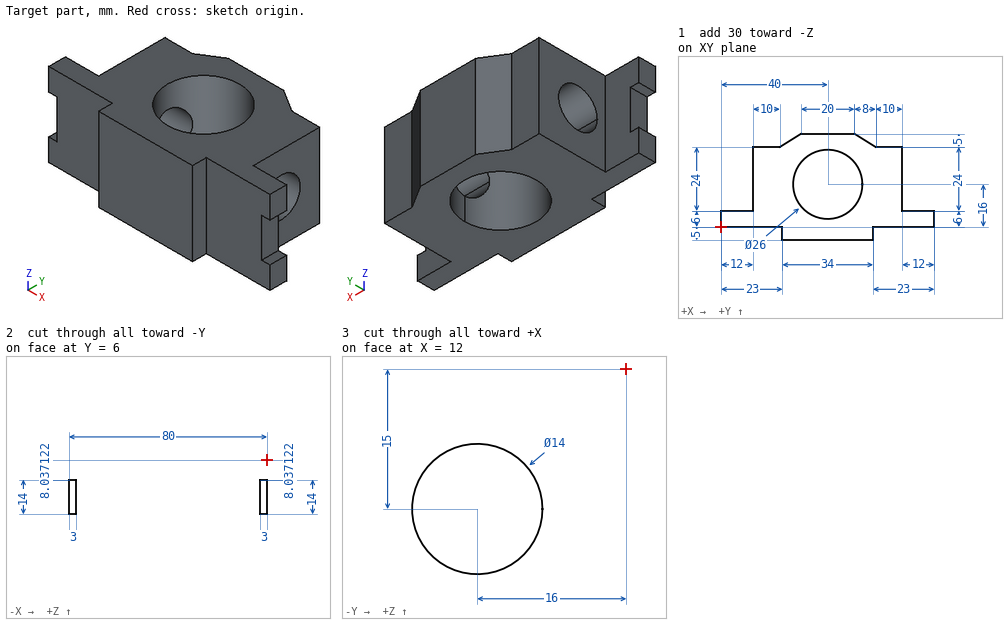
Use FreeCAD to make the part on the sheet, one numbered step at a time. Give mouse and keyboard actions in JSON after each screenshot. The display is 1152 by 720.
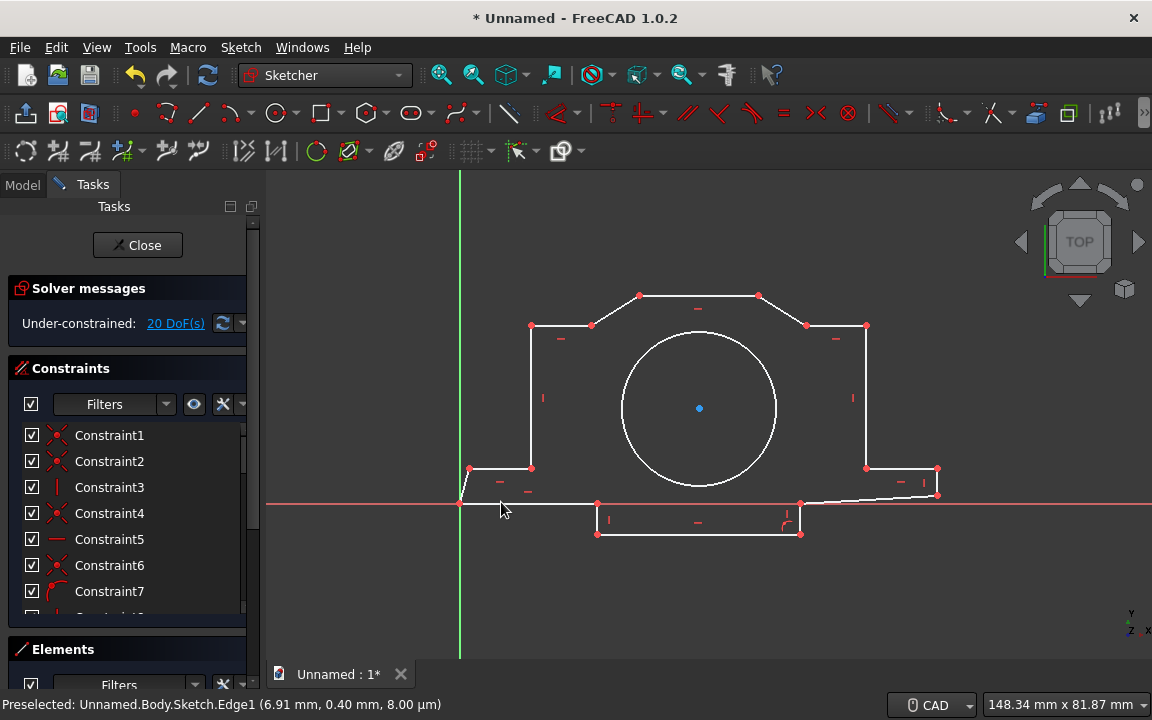
{"action": "left_click", "coordinate": [841, 502]}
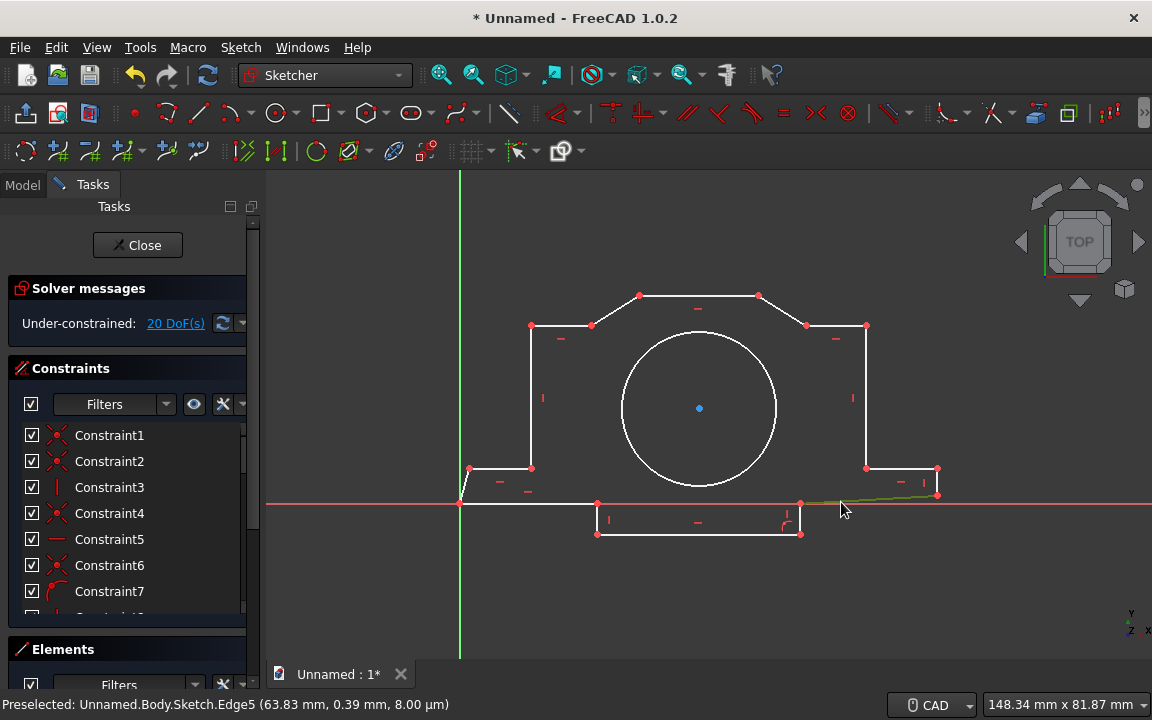
{"action": "key", "text": "h"}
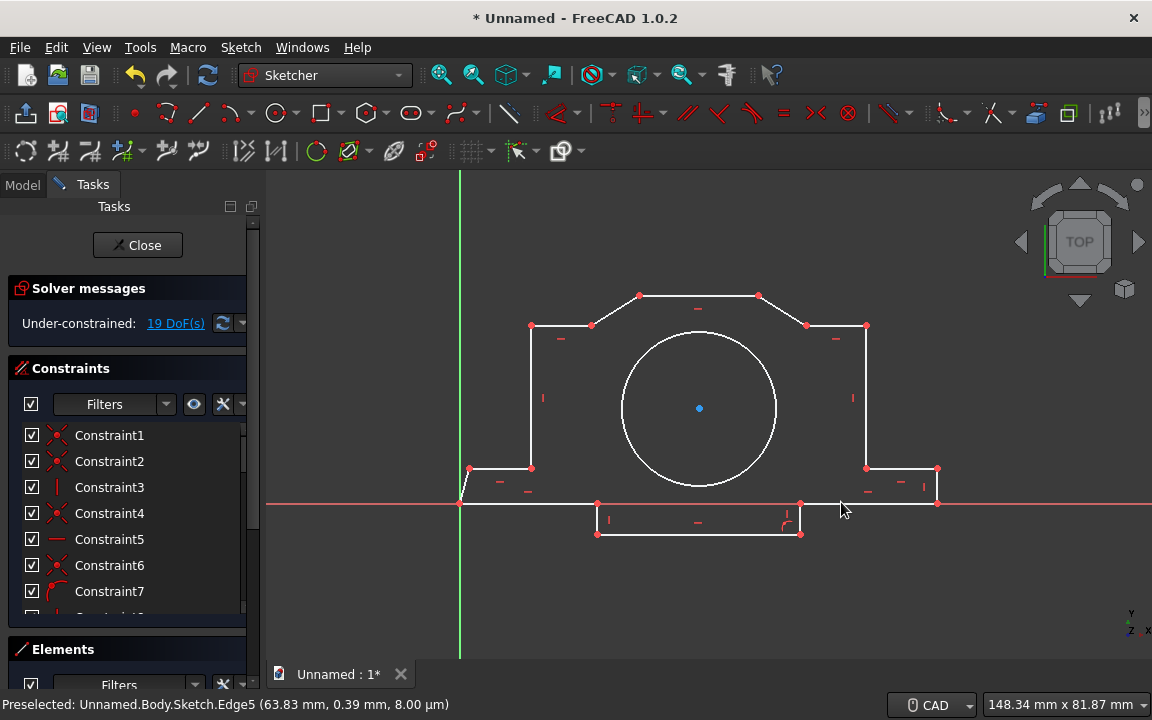
{"action": "scroll", "coordinate": [462, 493], "scroll_direction": "up", "scroll_amount": 2}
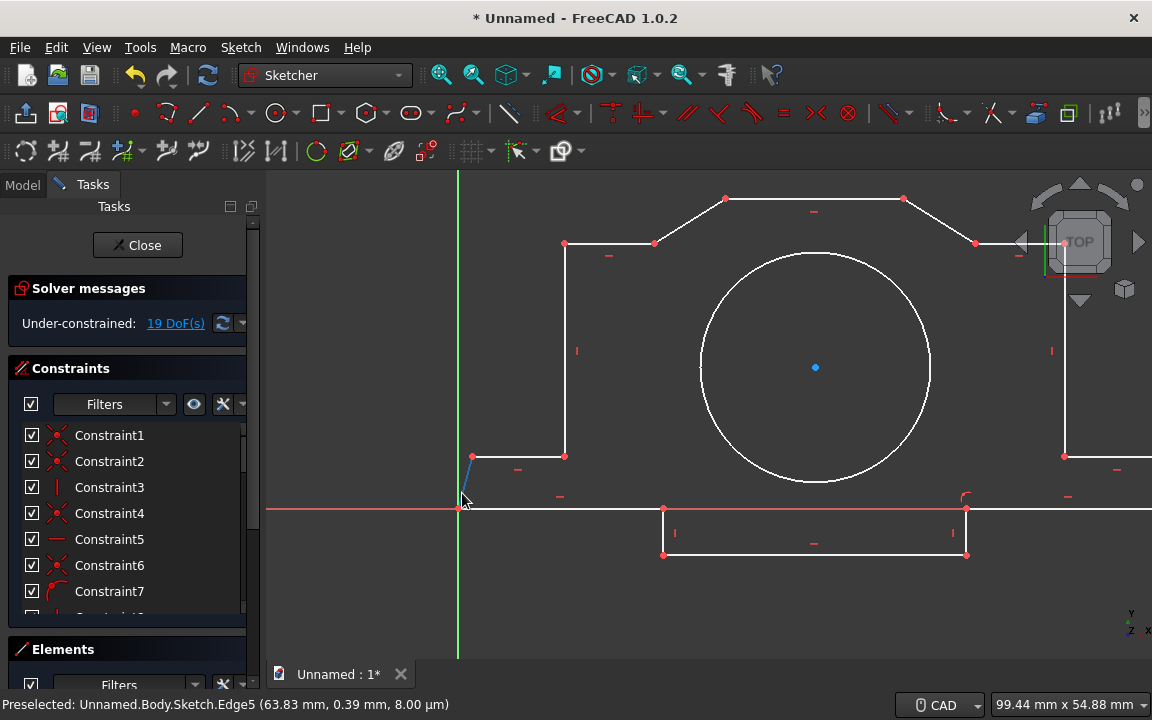
{"action": "left_click", "coordinate": [463, 493]}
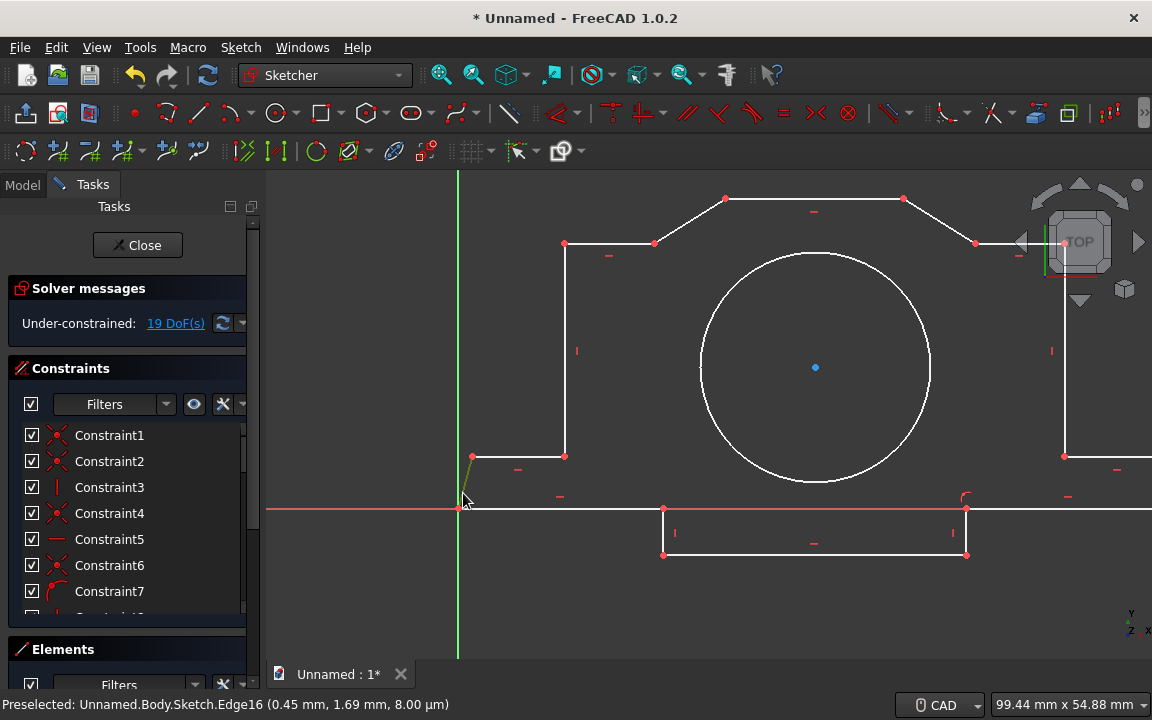
{"action": "key", "text": "v"}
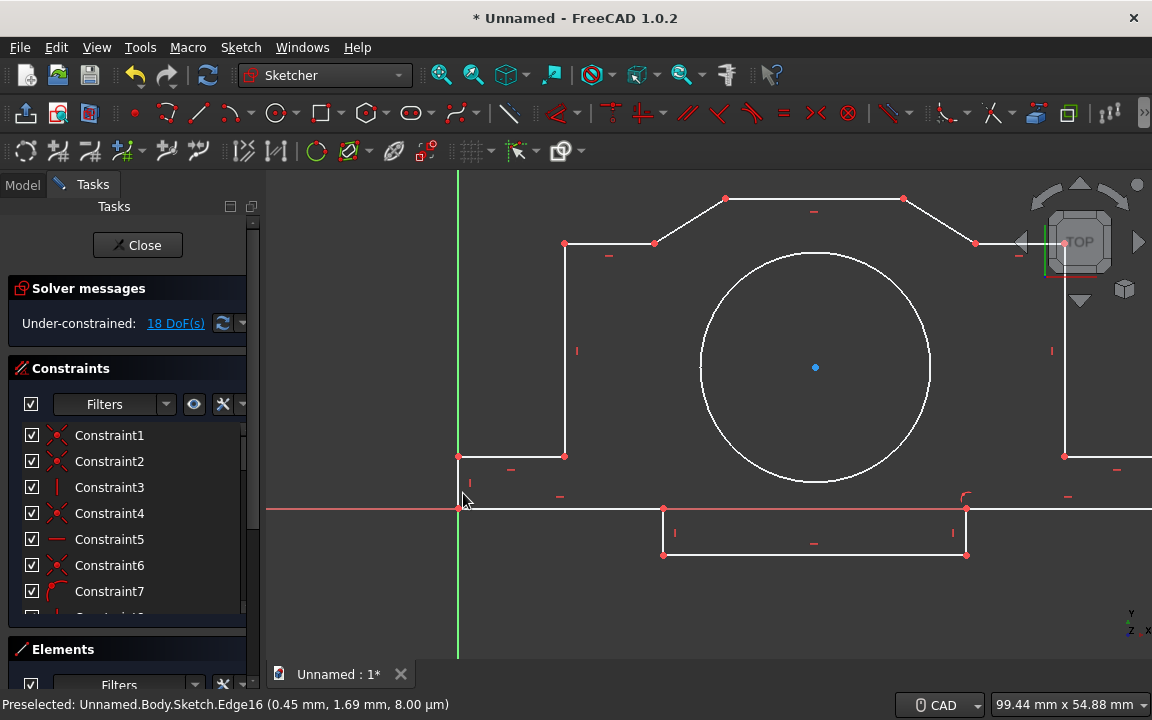
{"action": "left_click", "coordinate": [556, 114]}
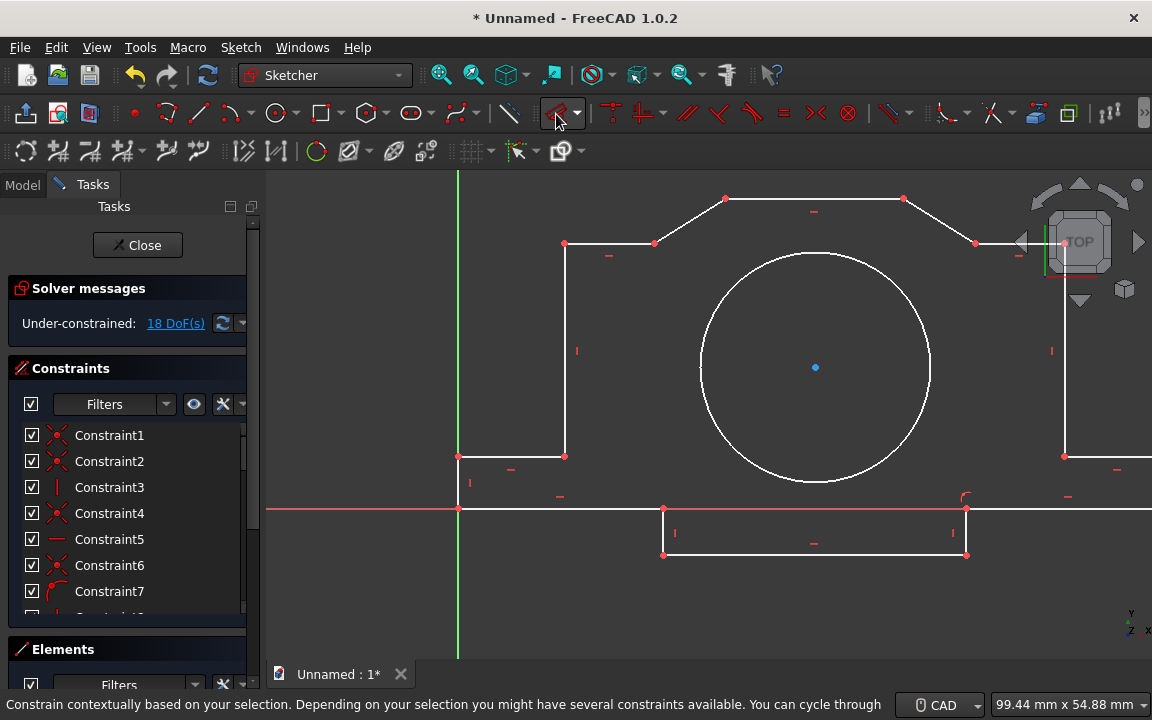
{"action": "left_click", "coordinate": [897, 286]}
{"action": "left_click", "coordinate": [920, 263]}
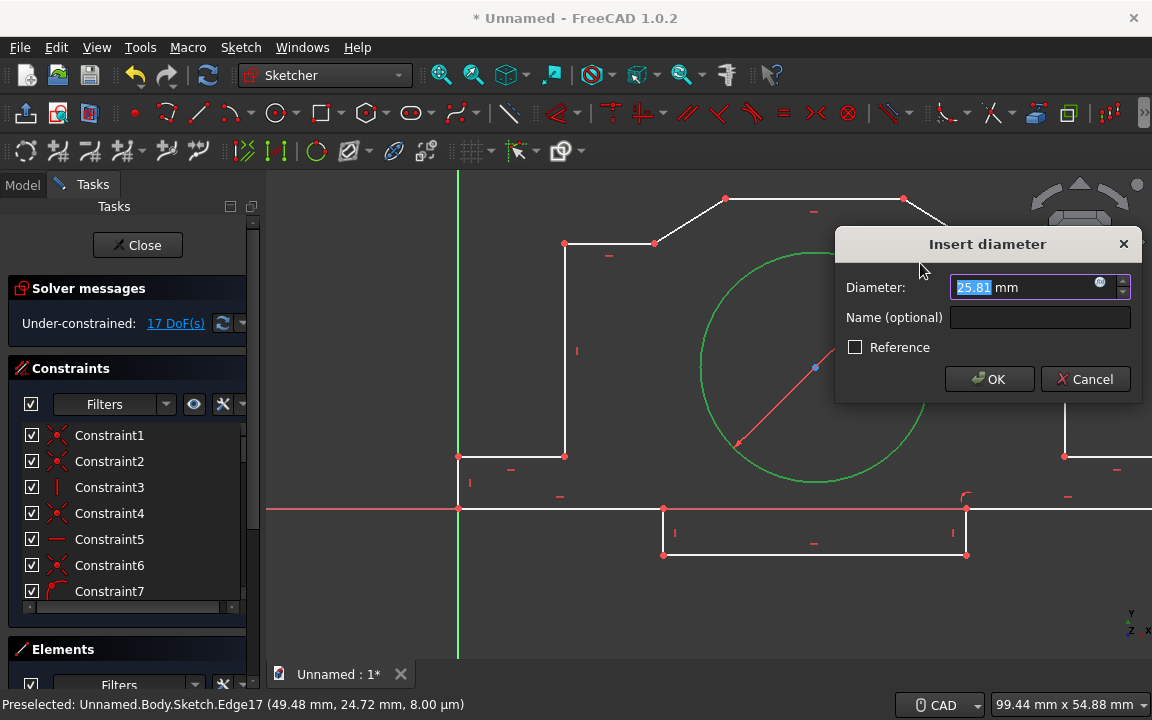
{"action": "type", "text": "26"}
{"action": "key", "text": "Return"}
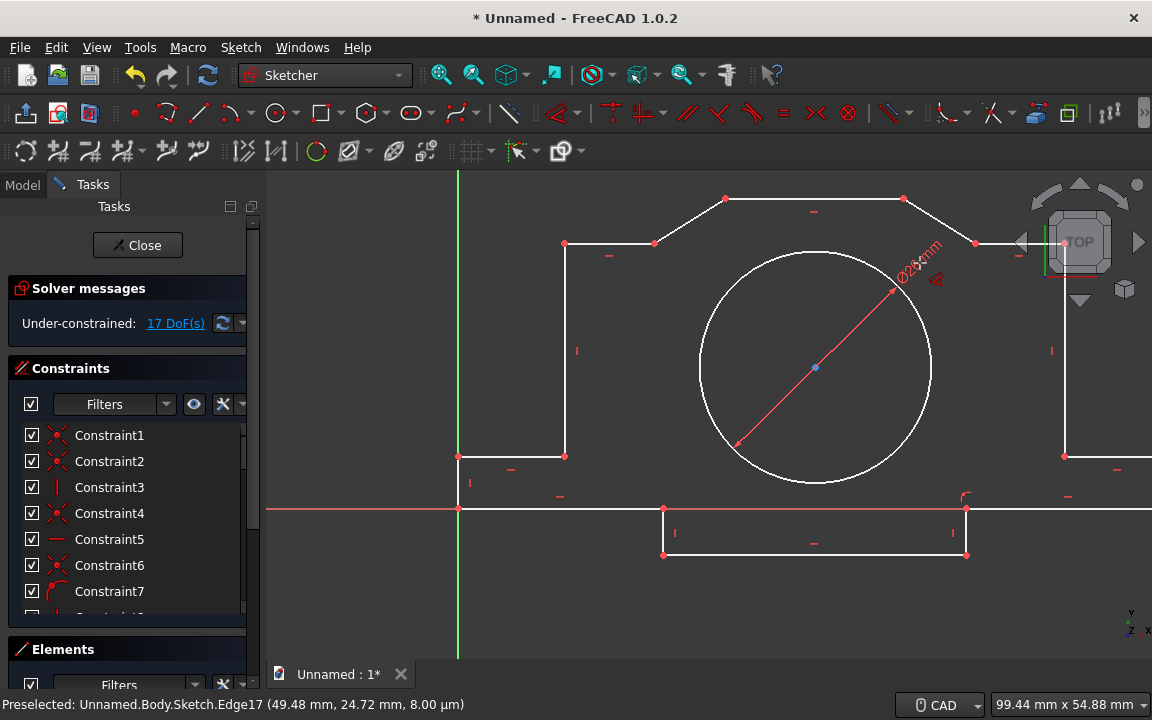
{"action": "left_click", "coordinate": [663, 523]}
{"action": "left_click", "coordinate": [629, 532]}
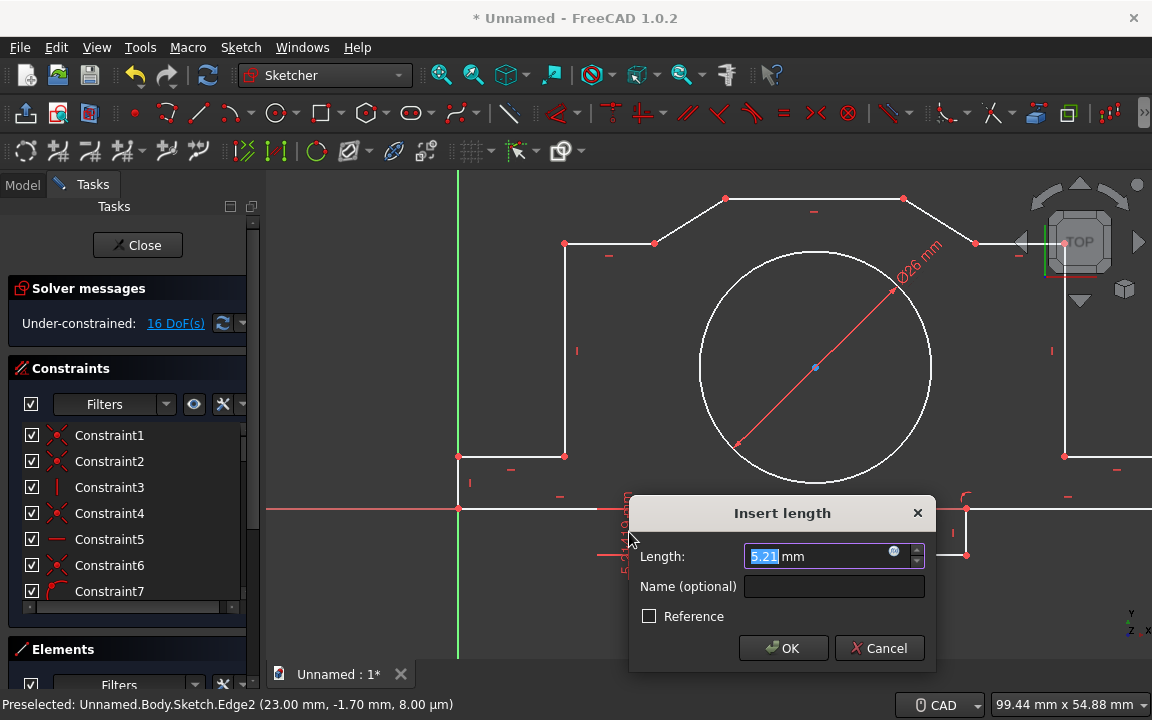
{"action": "type", "text": "5"}
{"action": "key", "text": "Return"}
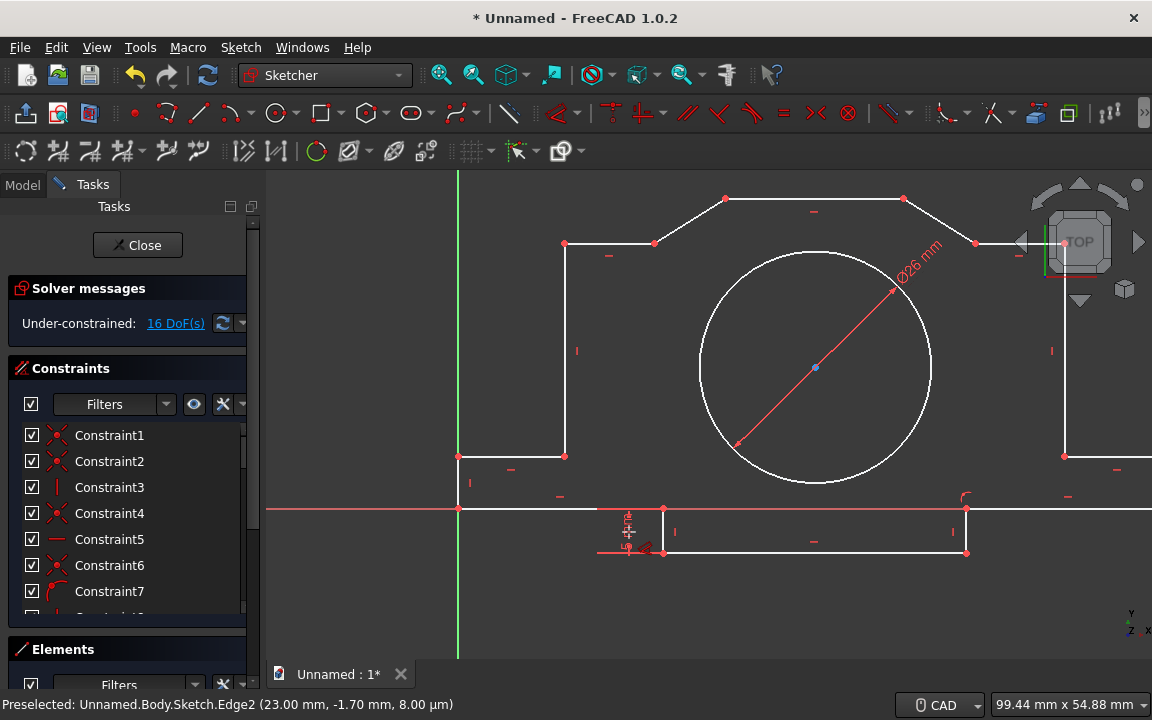
{"action": "scroll", "coordinate": [294, 494], "scroll_direction": "down", "scroll_amount": 2}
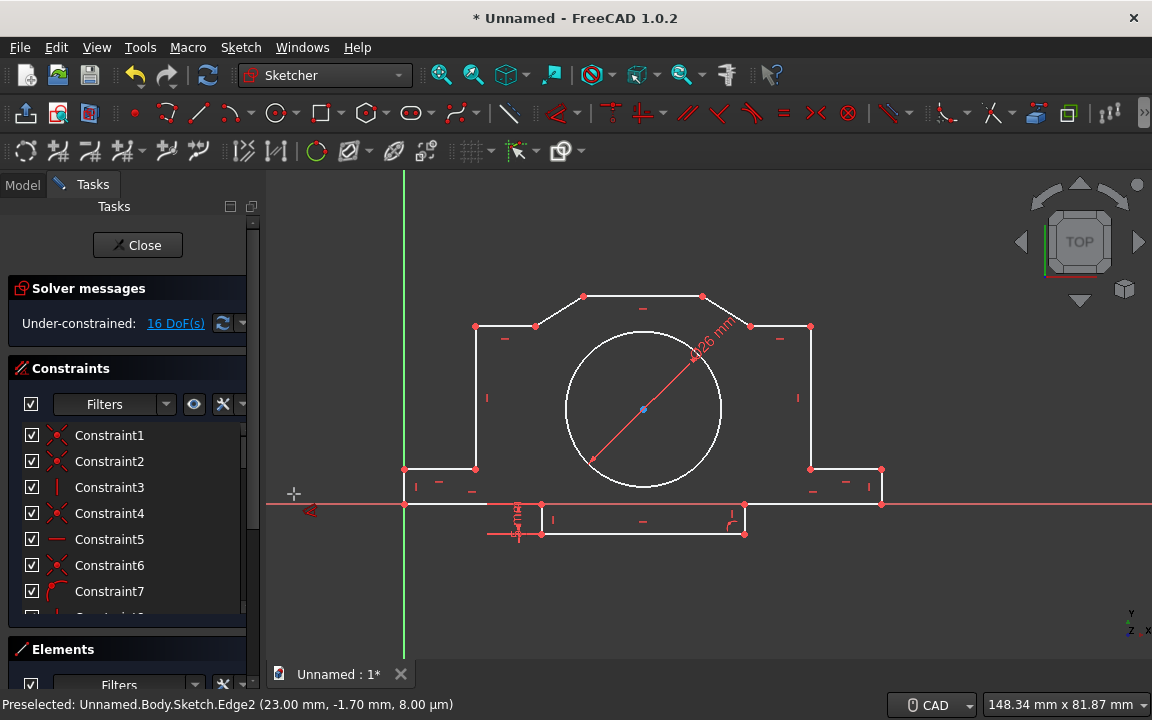
{"action": "scroll", "coordinate": [882, 494], "scroll_direction": "up", "scroll_amount": 2}